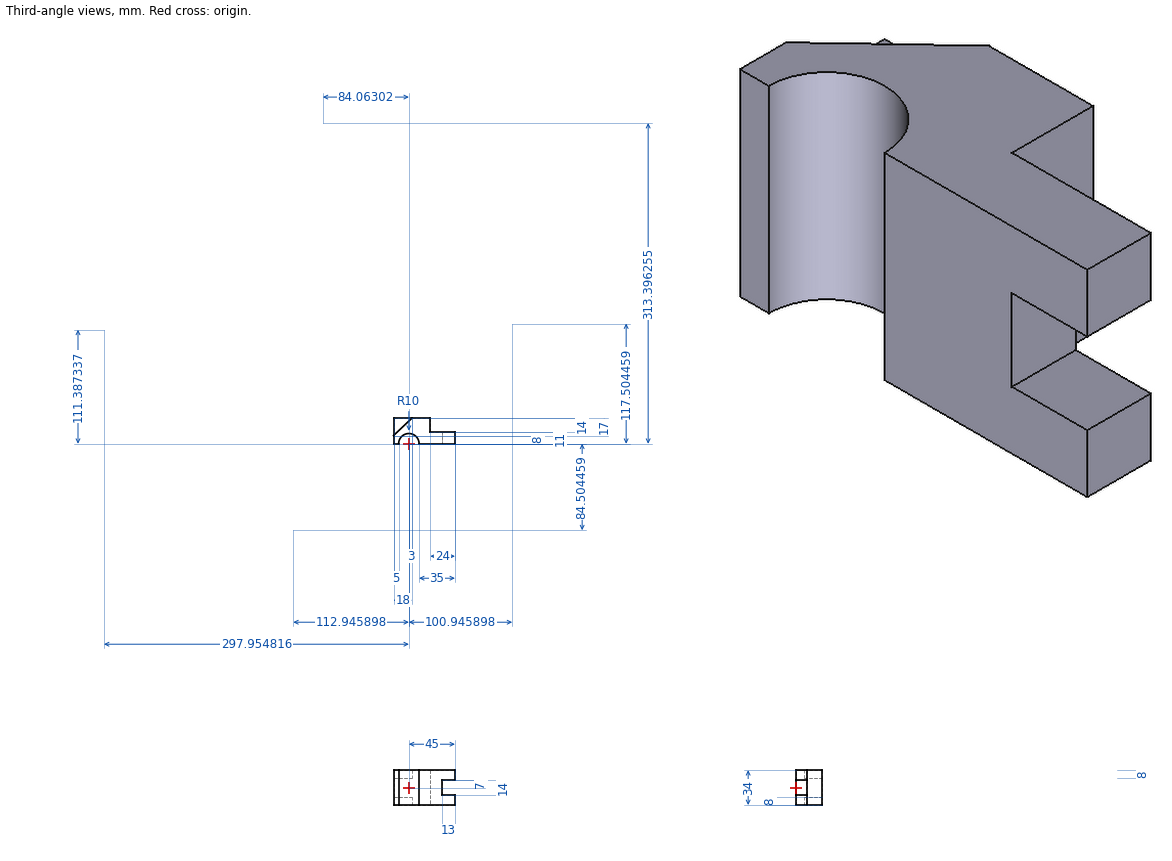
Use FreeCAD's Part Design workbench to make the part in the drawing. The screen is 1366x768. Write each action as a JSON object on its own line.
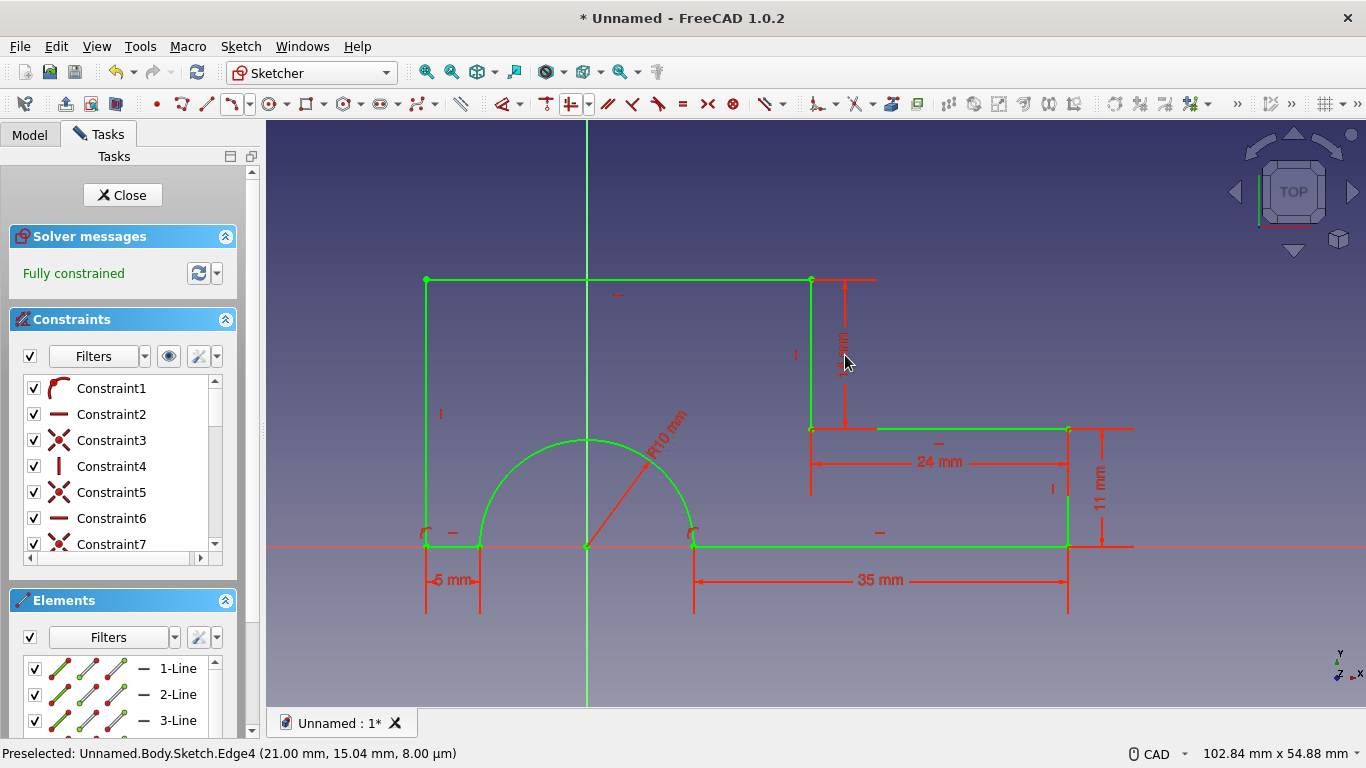
{"action": "left_click", "coordinate": [123, 195]}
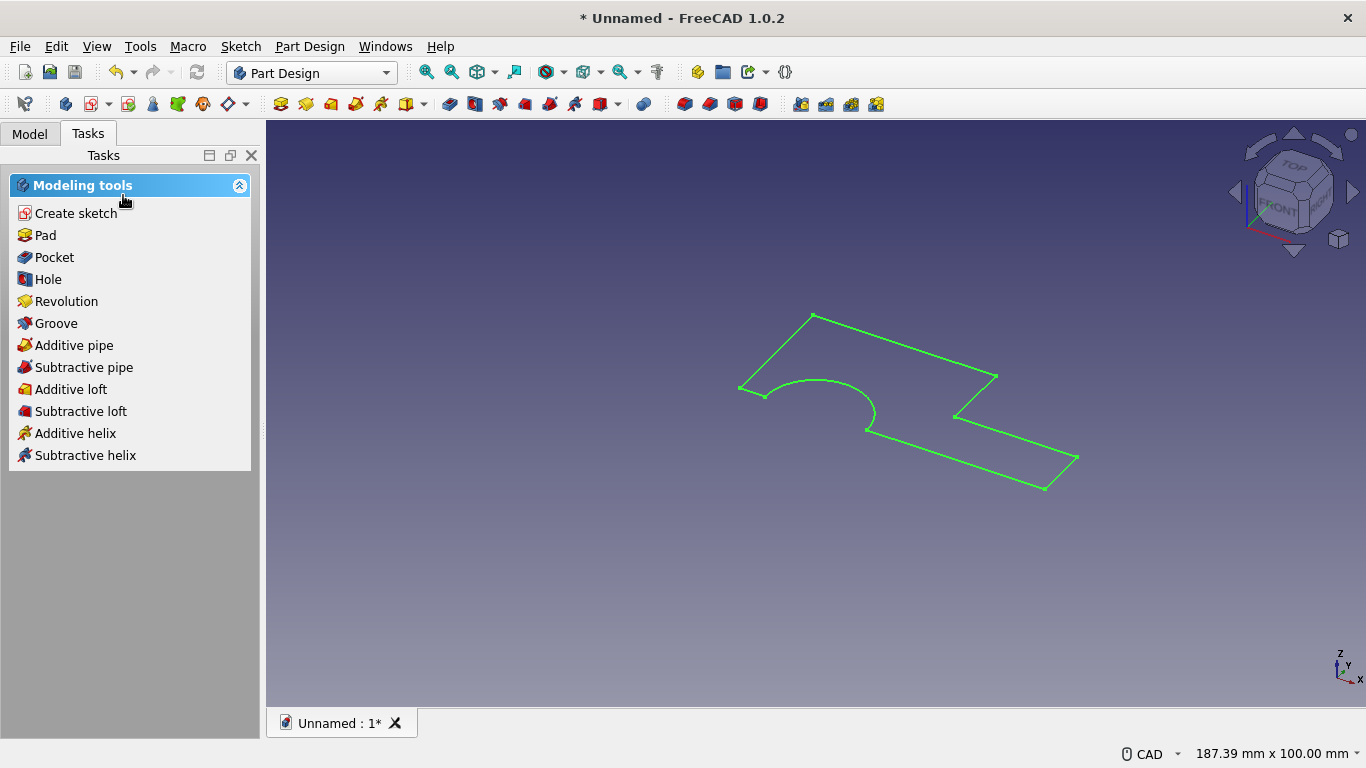
{"action": "left_click", "coordinate": [281, 104]}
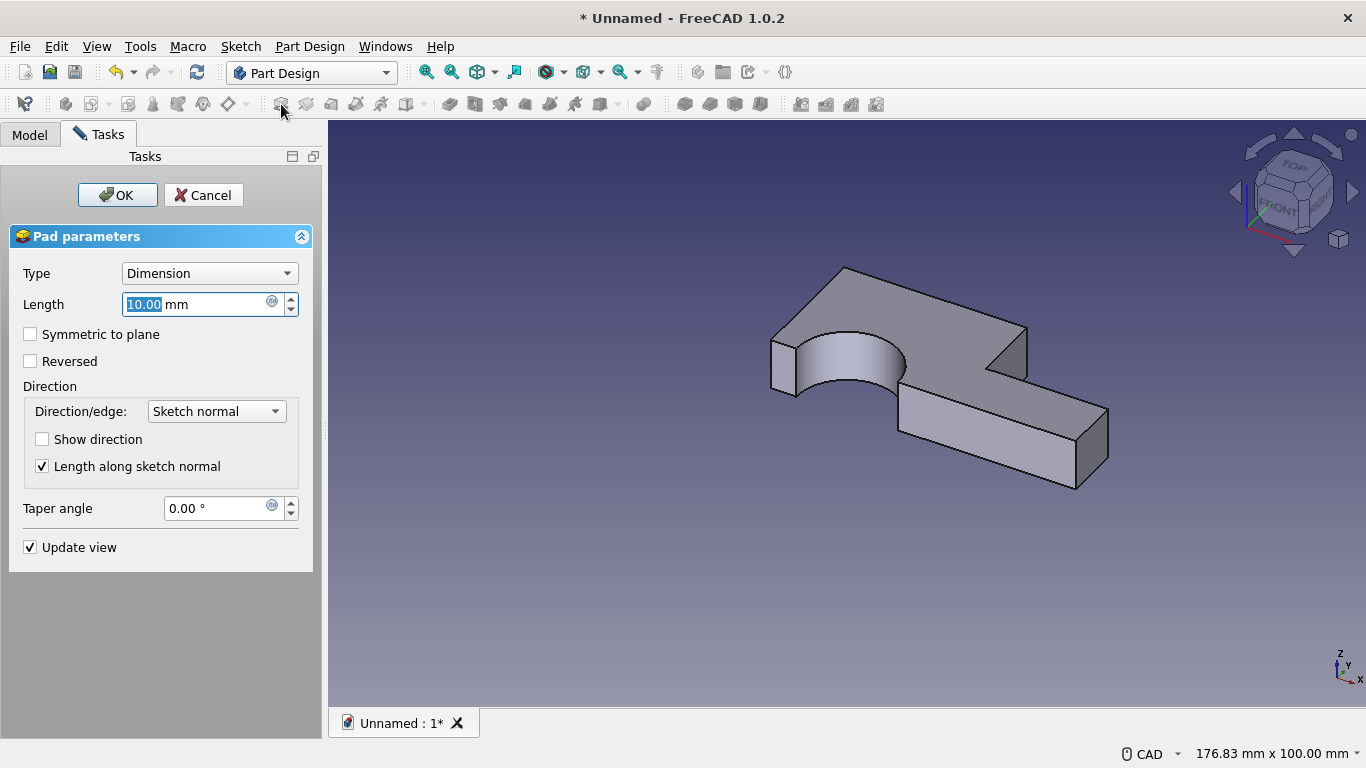
{"action": "type", "text": "34"}
{"action": "key", "text": "Tab"}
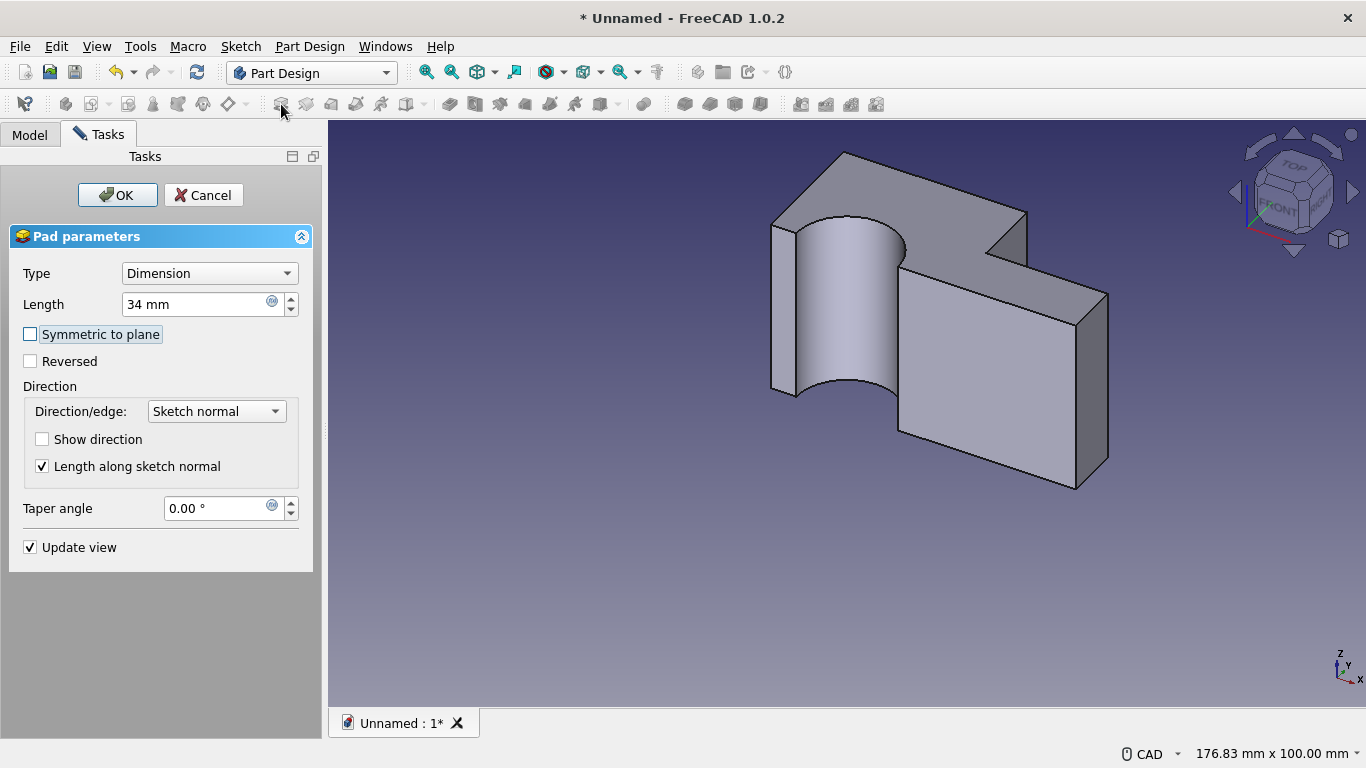
{"action": "left_click", "coordinate": [31, 334]}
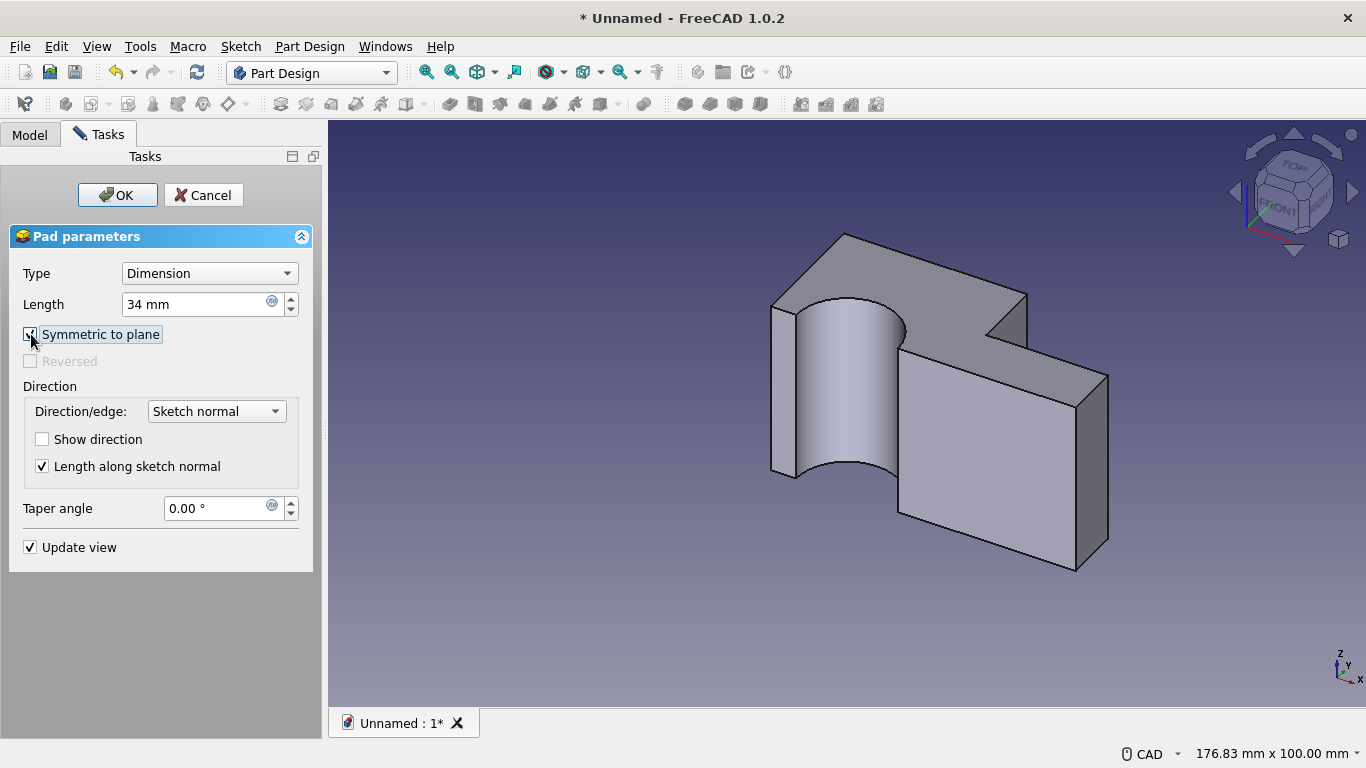
{"action": "left_click", "coordinate": [118, 195]}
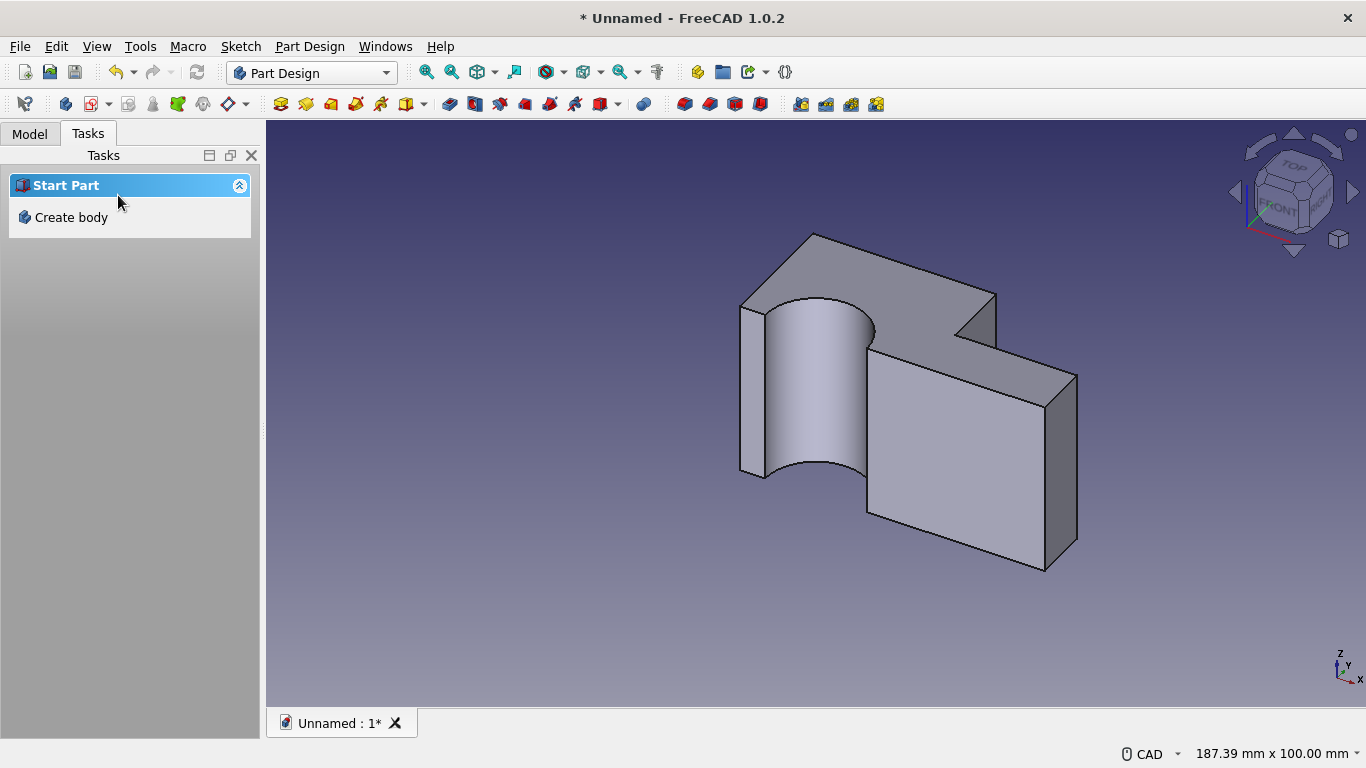
{"action": "key", "text": "4"}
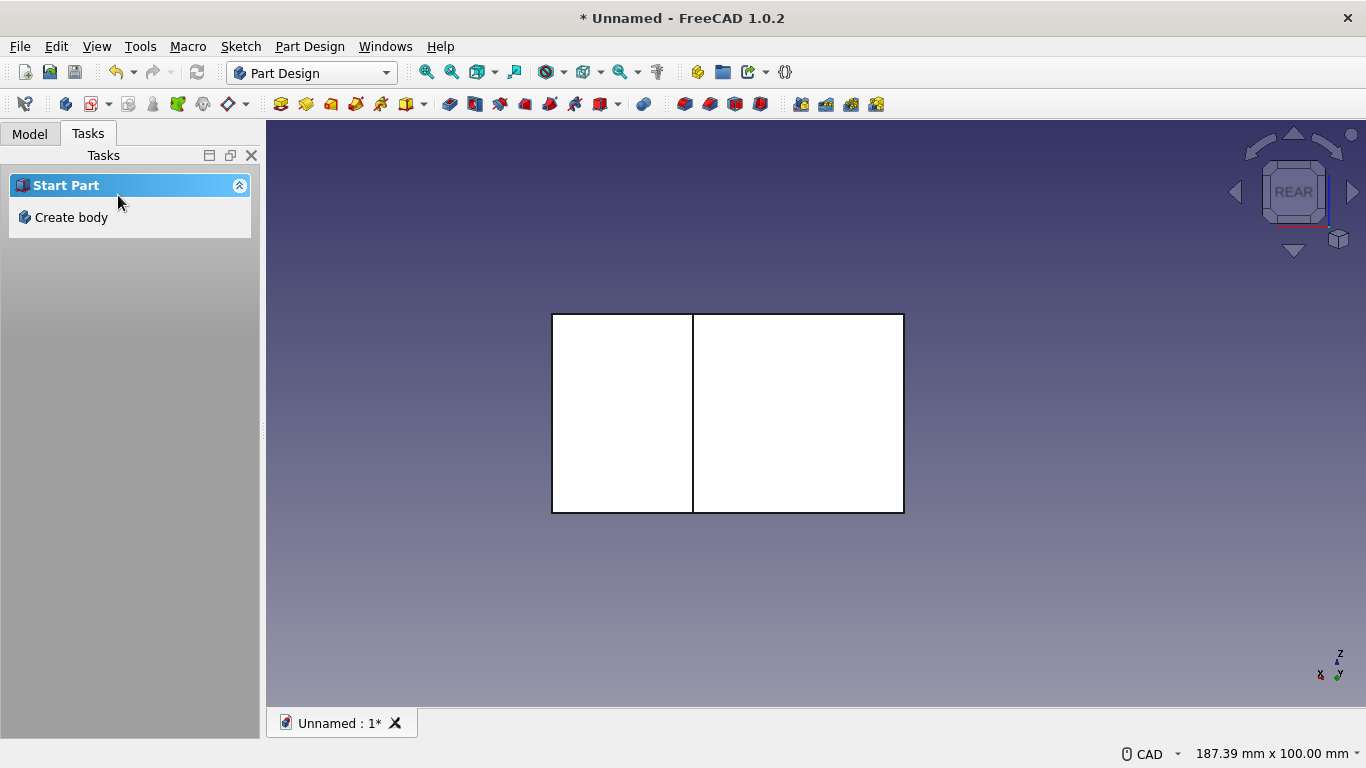
{"action": "left_click", "coordinate": [427, 72]}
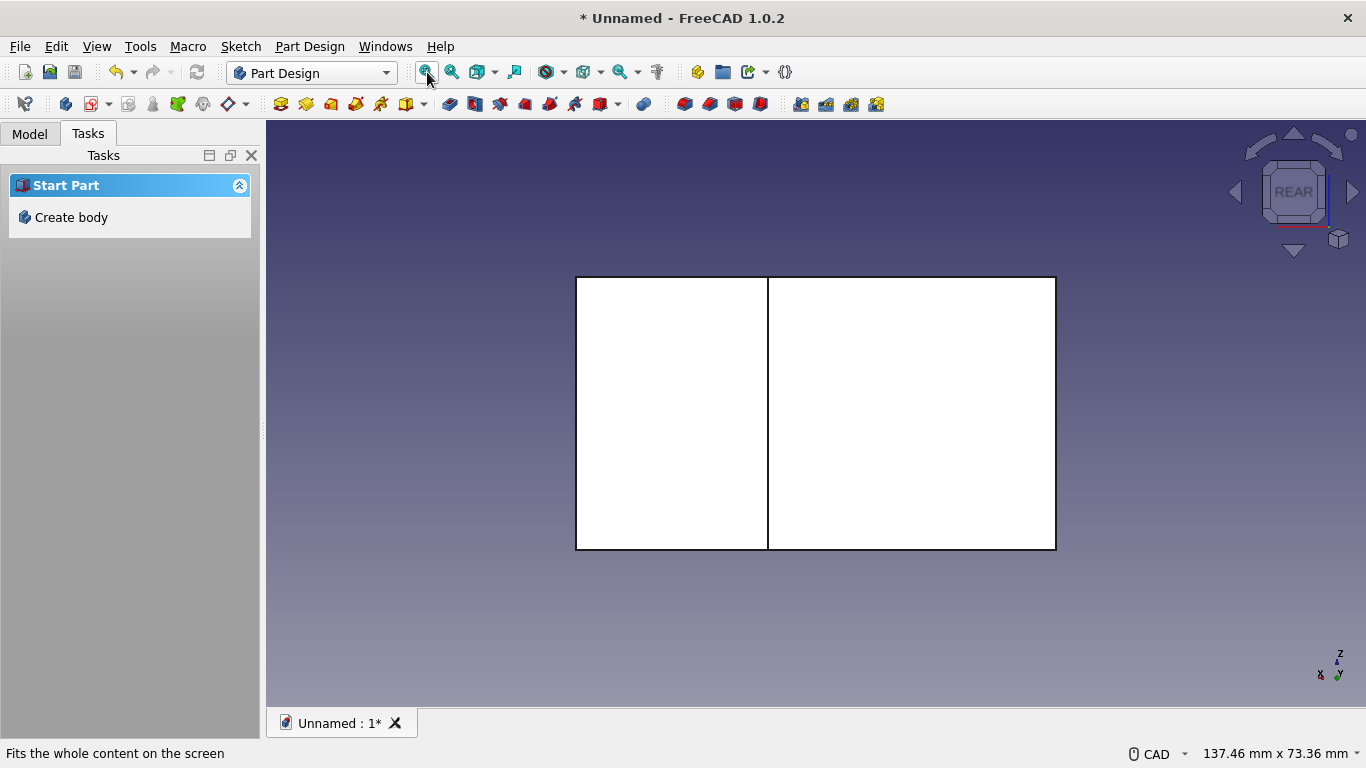
{"action": "left_click", "coordinate": [672, 374]}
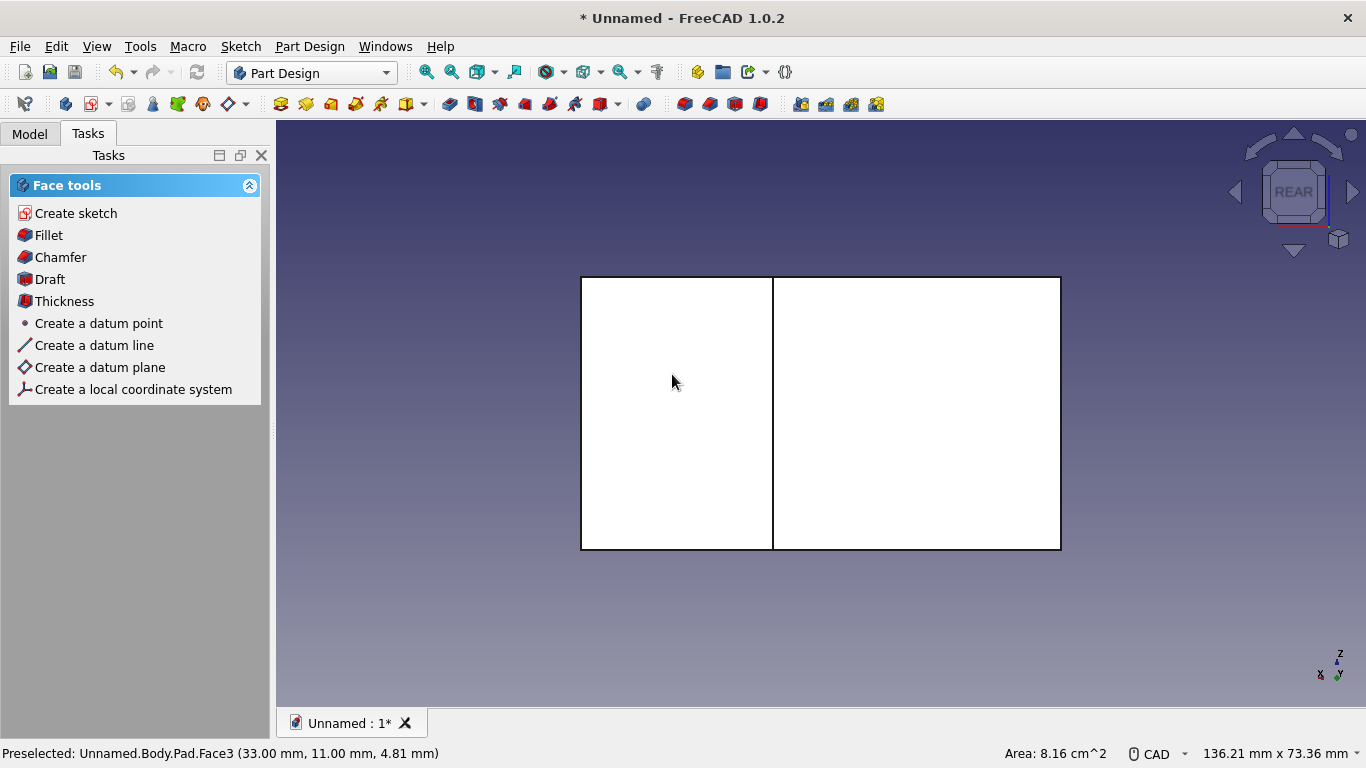
{"action": "left_click", "coordinate": [90, 104]}